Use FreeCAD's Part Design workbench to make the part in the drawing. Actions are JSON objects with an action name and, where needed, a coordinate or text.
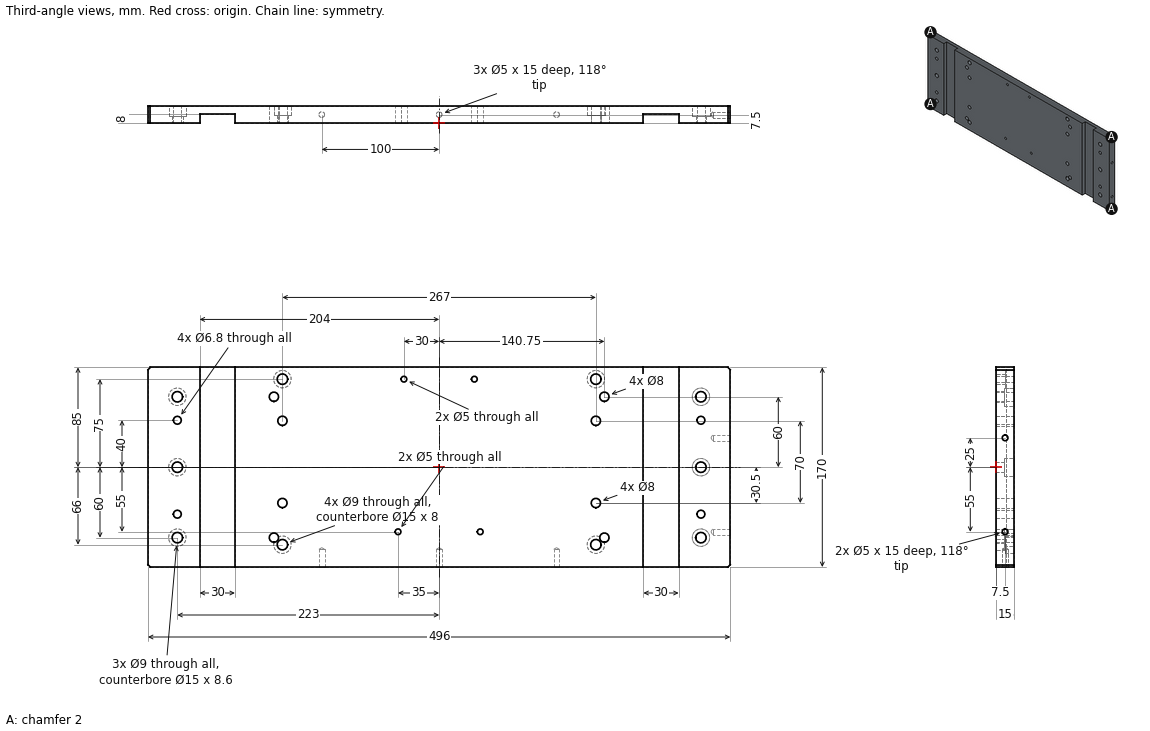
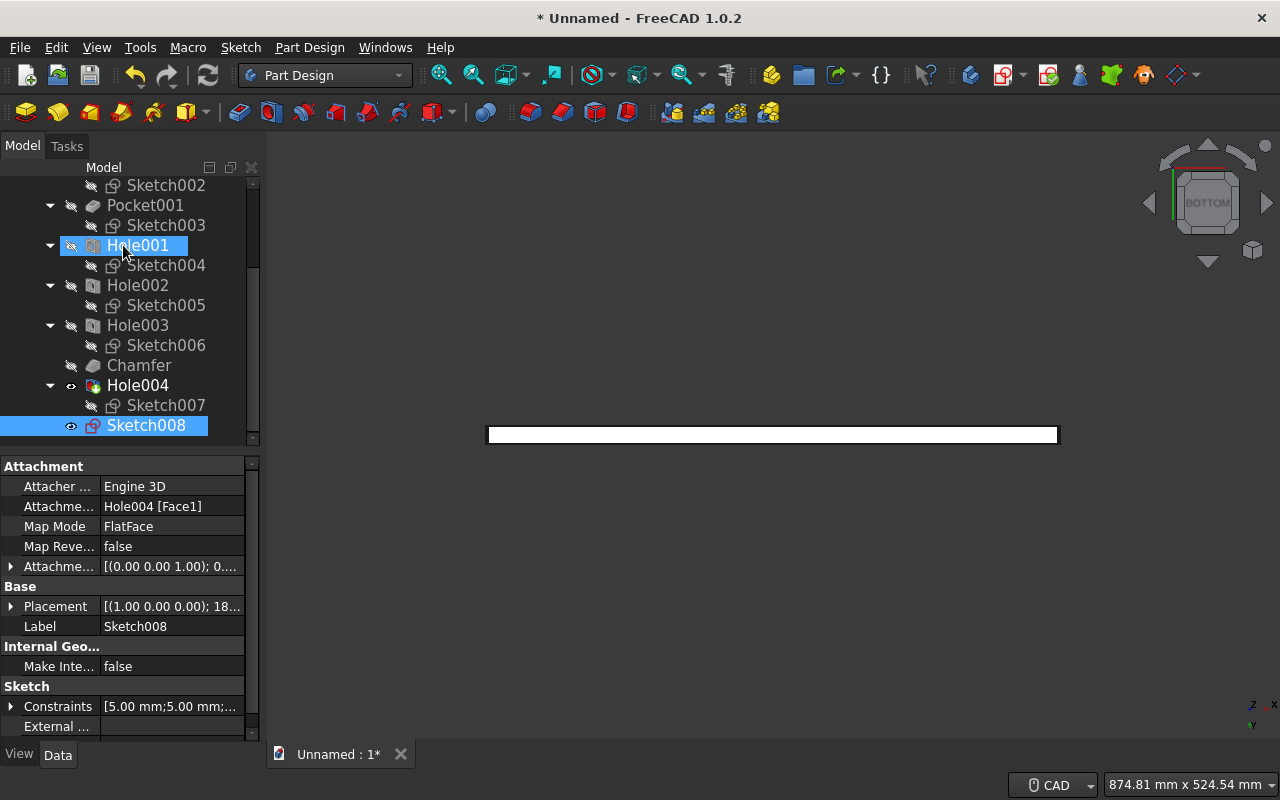
{"action": "left_click", "coordinate": [272, 112]}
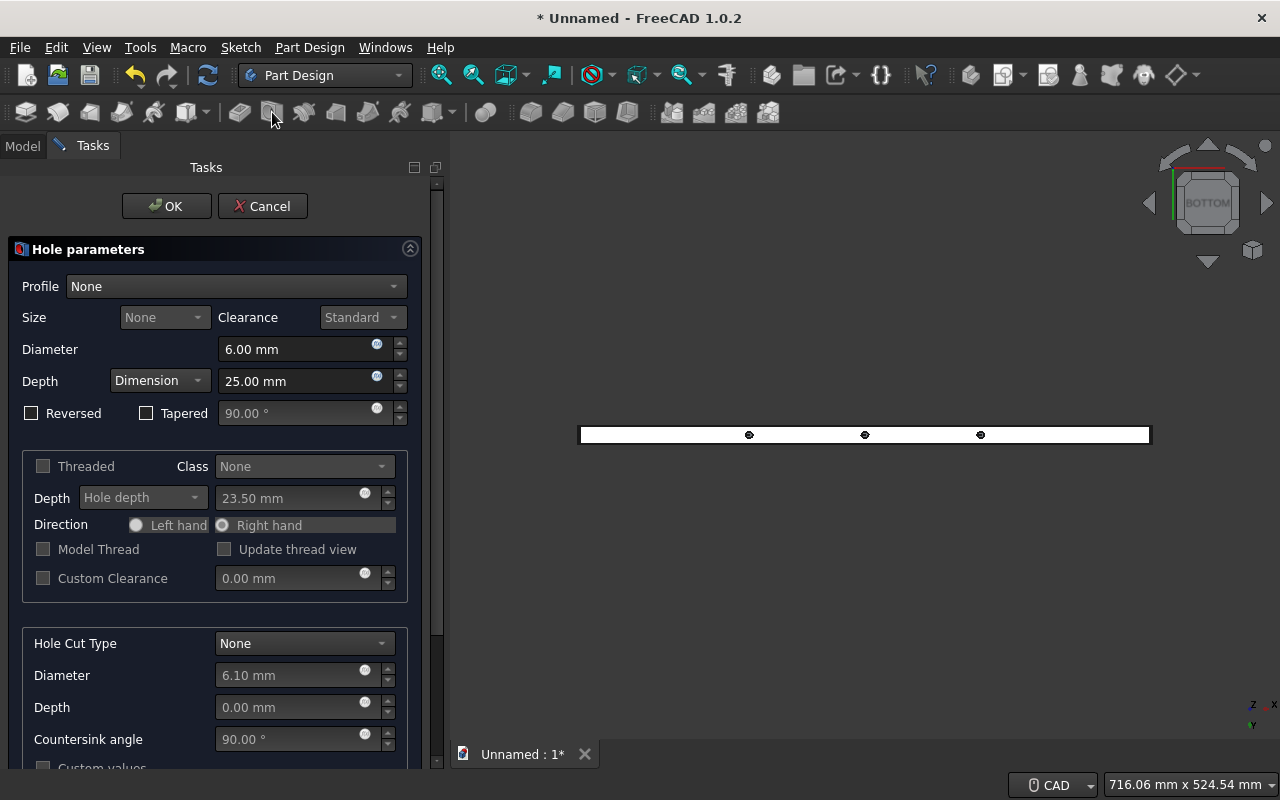
{"action": "triple_click", "coordinate": [305, 349]}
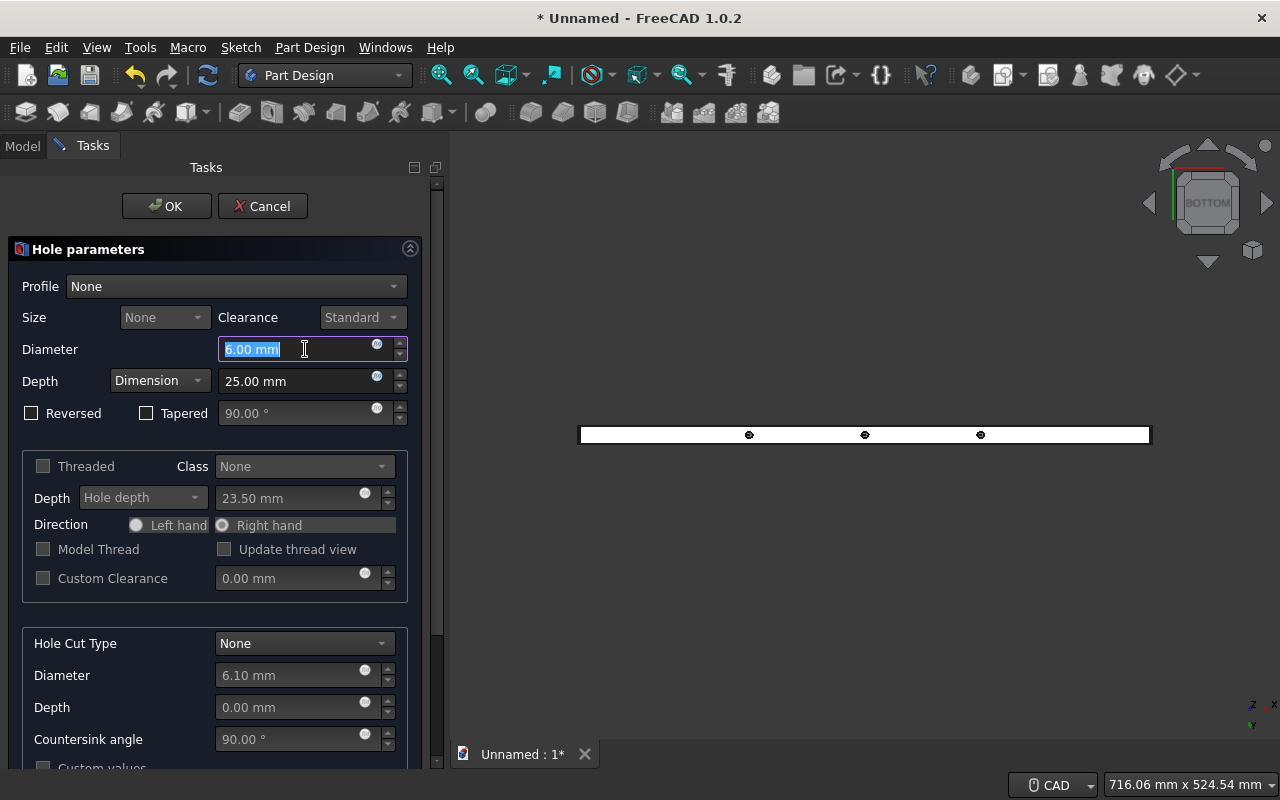
{"action": "type", "text": "5"}
{"action": "key", "text": "Tab"}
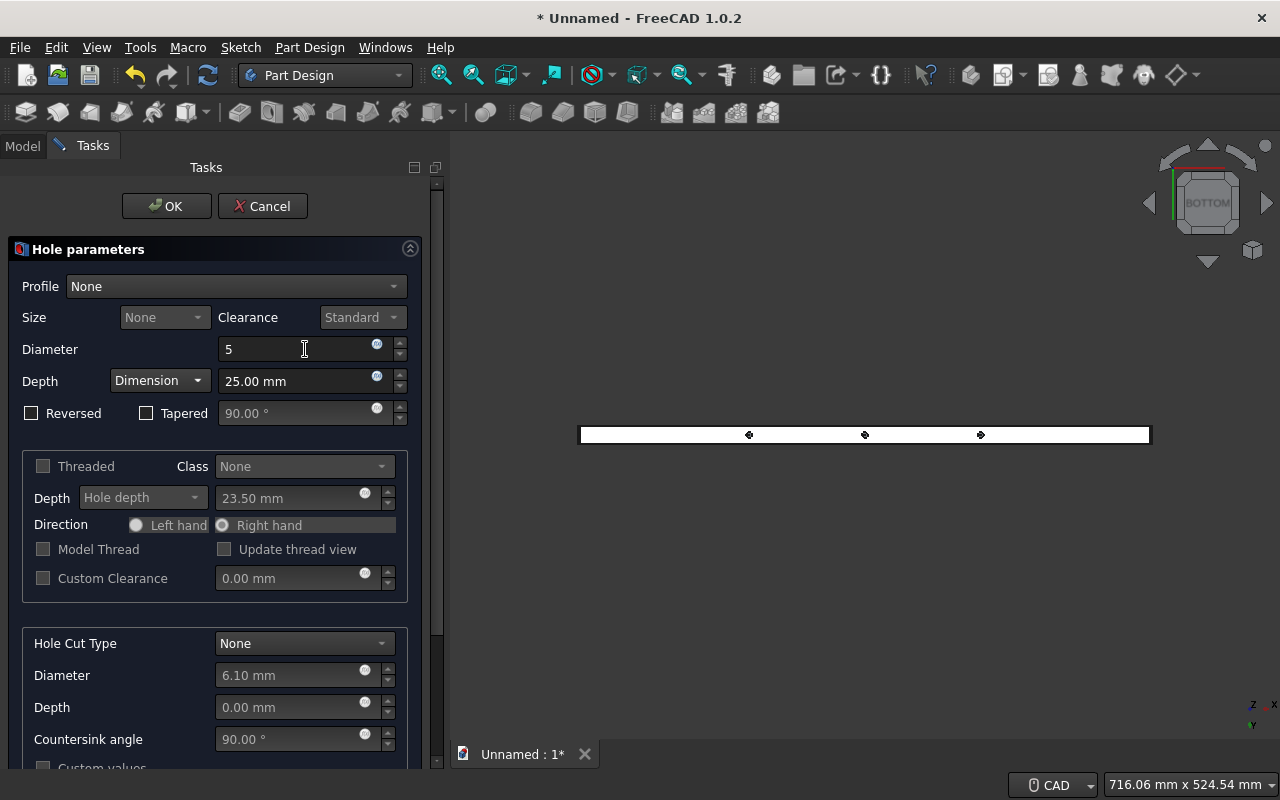
{"action": "triple_click", "coordinate": [305, 381]}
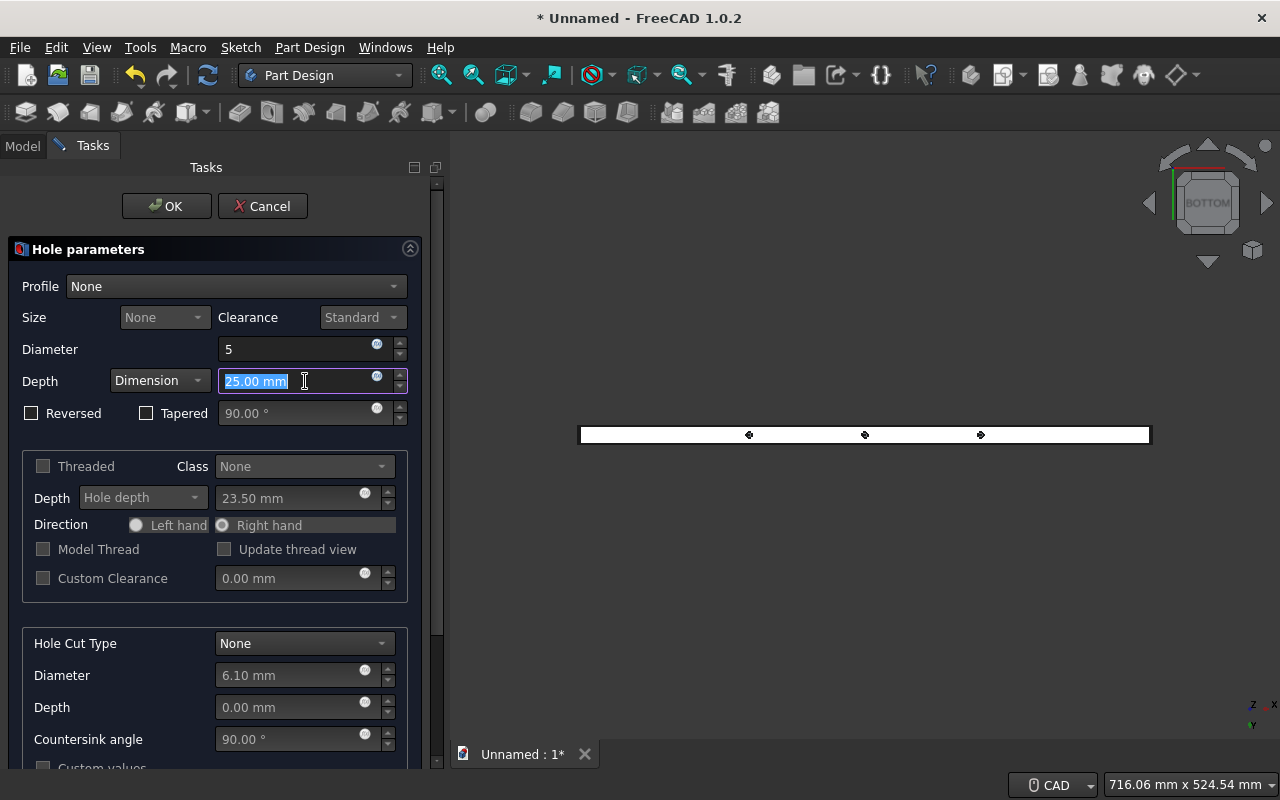
{"action": "type", "text": "15"}
{"action": "key", "text": "Tab"}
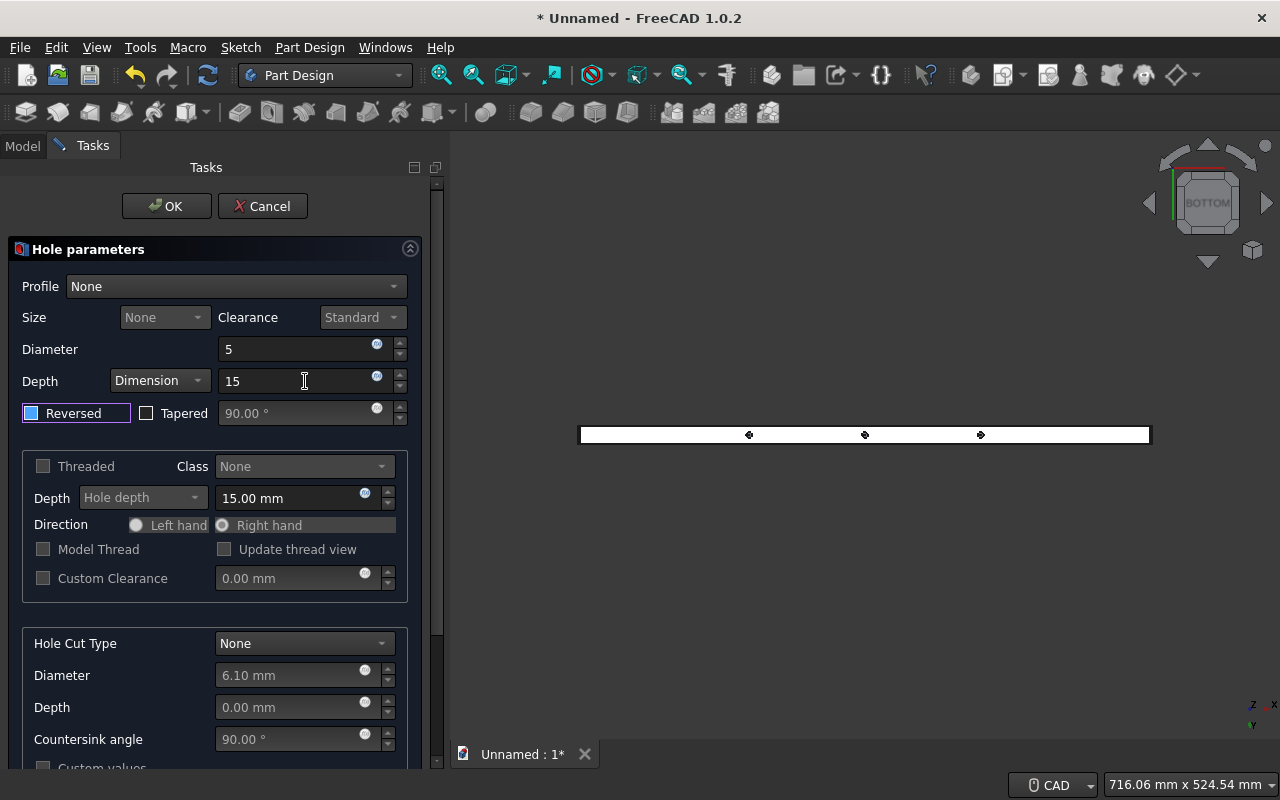
{"action": "left_click", "coordinate": [167, 206]}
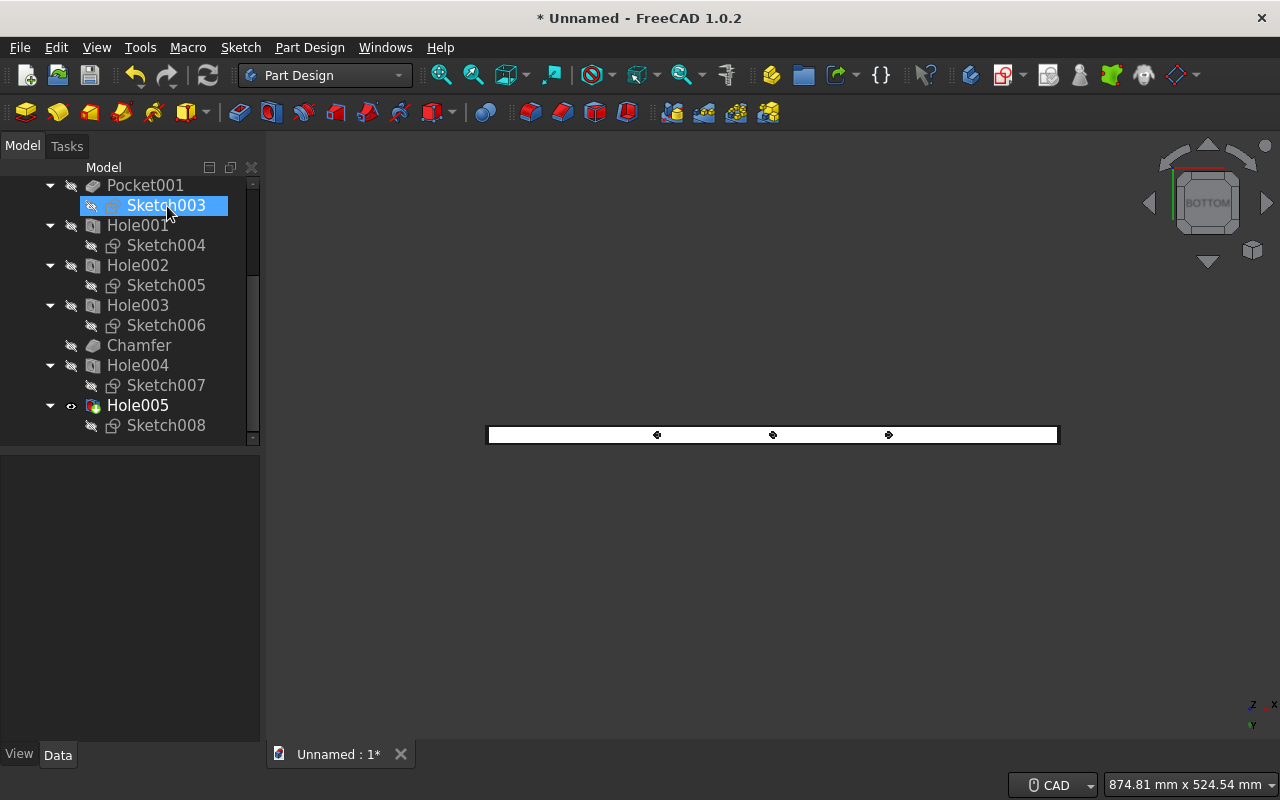
{"action": "scroll", "coordinate": [140, 301], "scroll_direction": "down", "scroll_amount": 3}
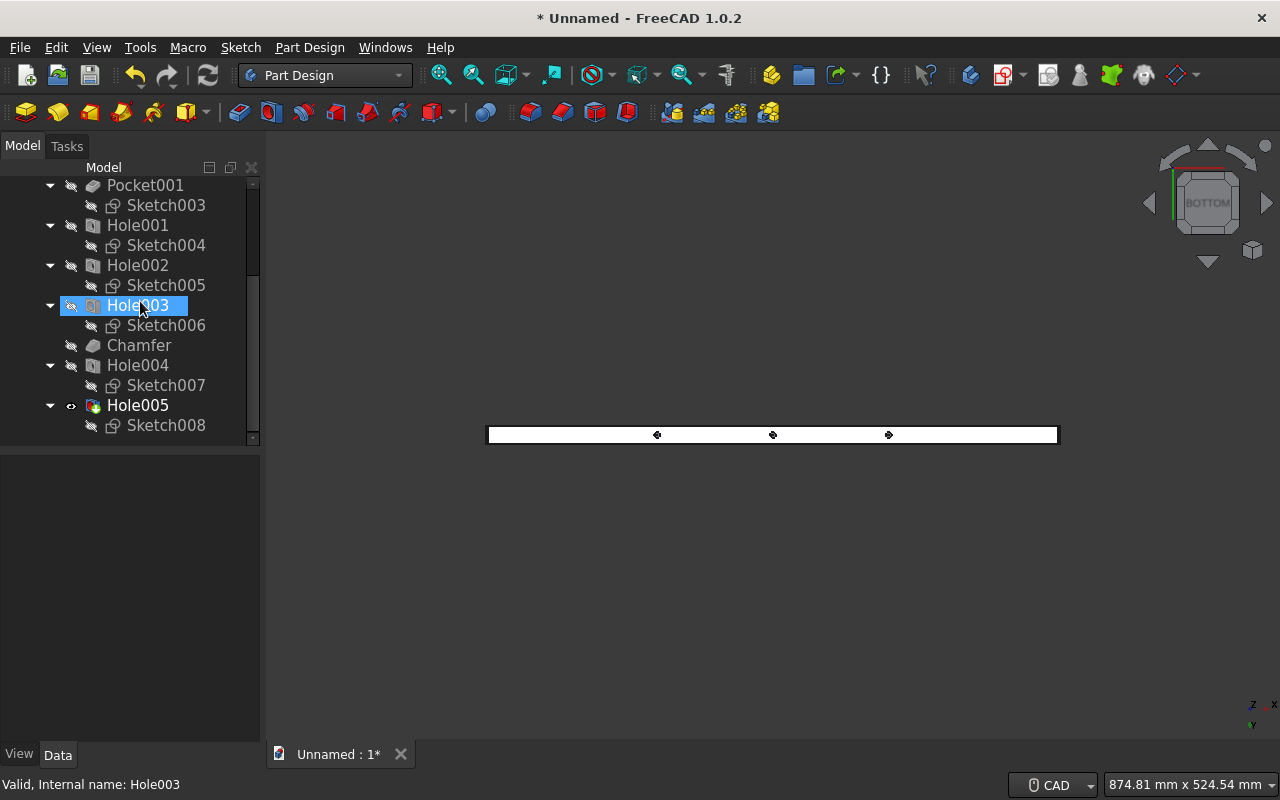
{"action": "scroll", "coordinate": [140, 301], "scroll_direction": "up", "scroll_amount": 15}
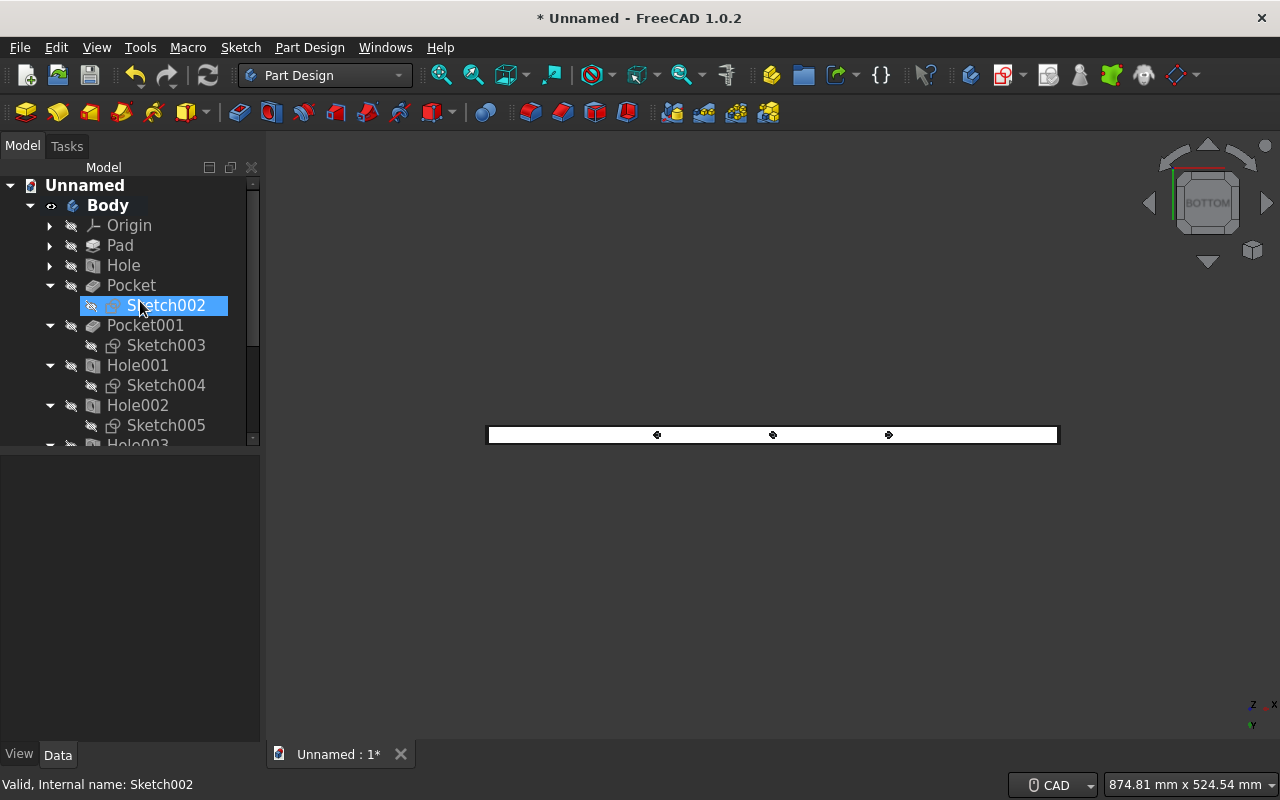
{"action": "left_click", "coordinate": [116, 266]}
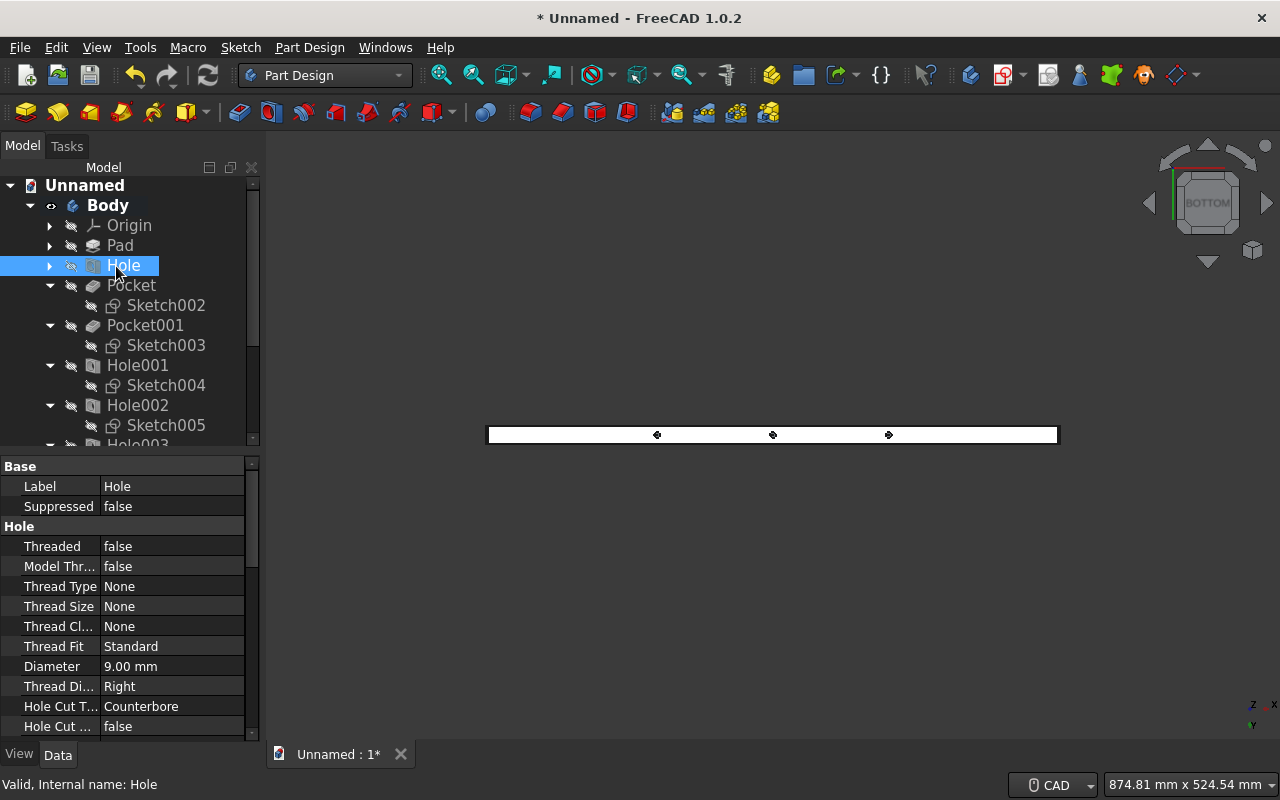
{"action": "left_click", "coordinate": [672, 112]}